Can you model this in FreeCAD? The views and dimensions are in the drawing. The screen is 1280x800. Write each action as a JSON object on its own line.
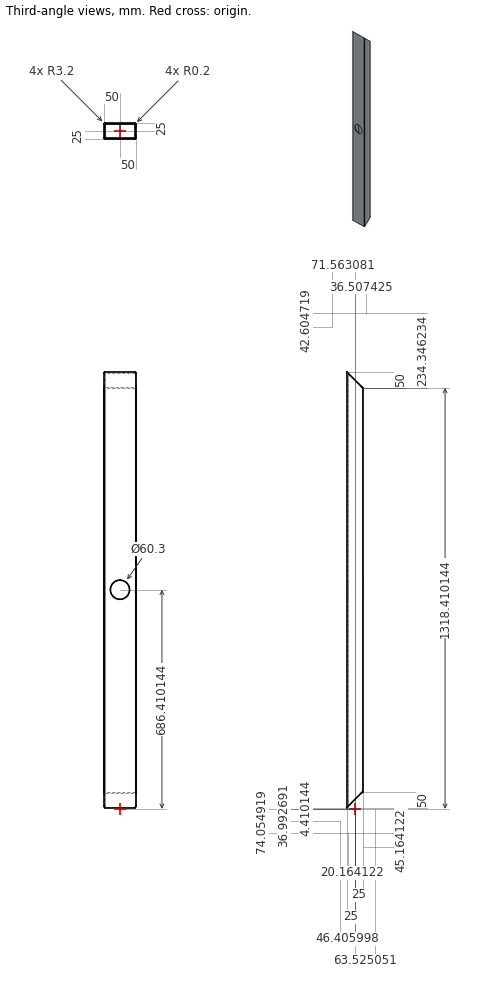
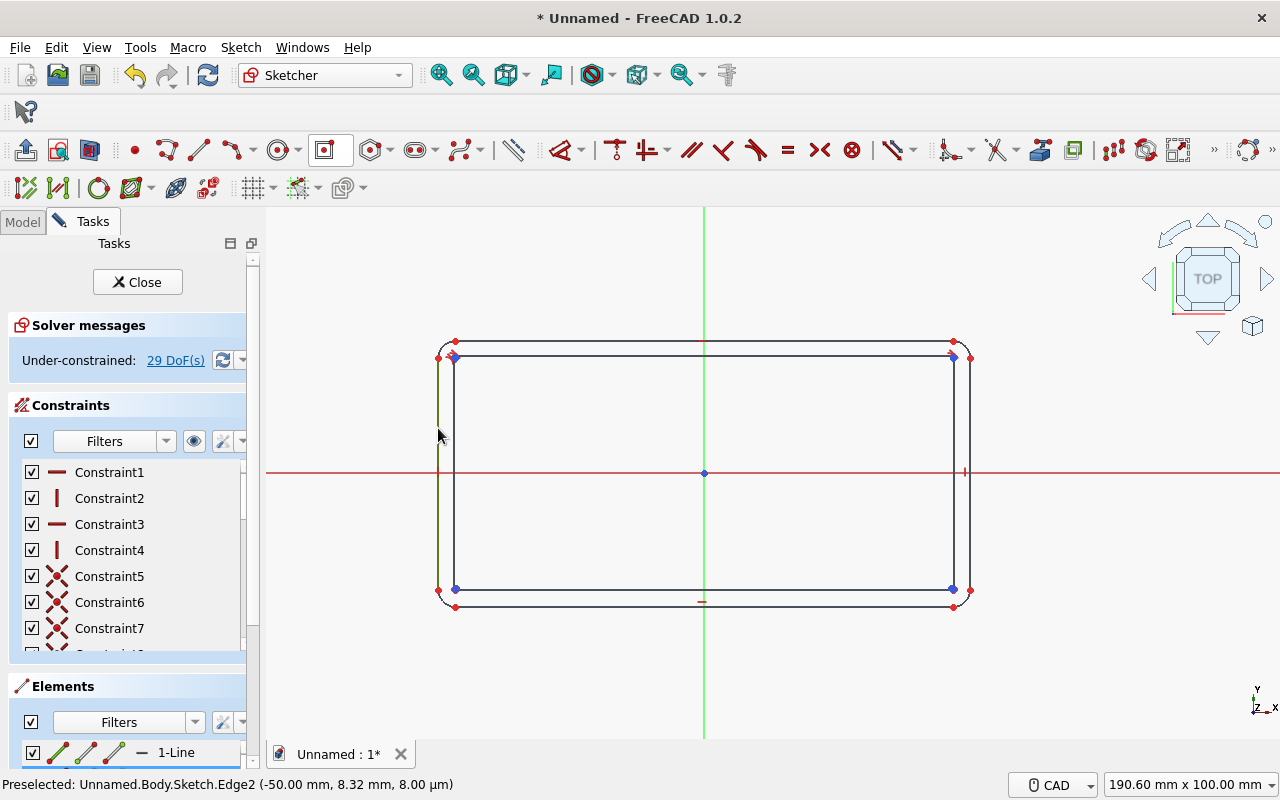
{"action": "left_click", "coordinate": [444, 602]}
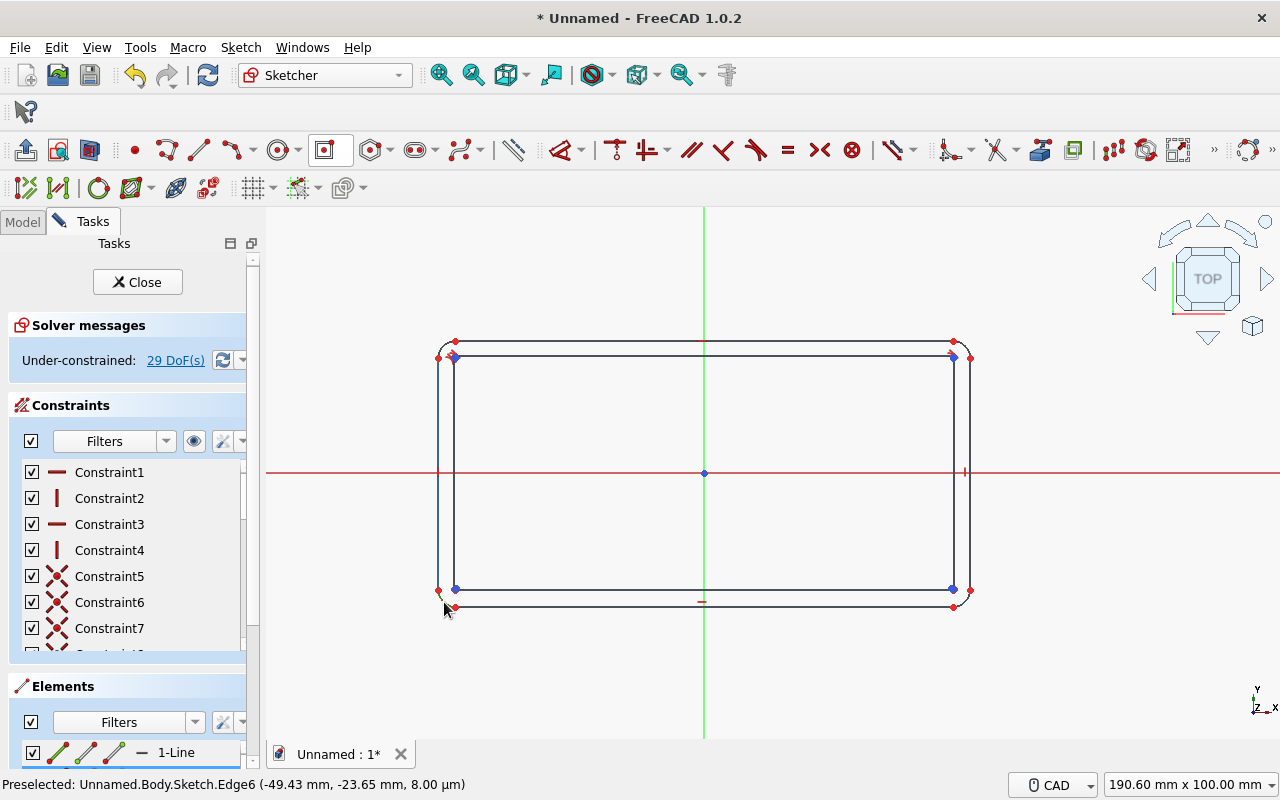
{"action": "left_click", "coordinate": [756, 150]}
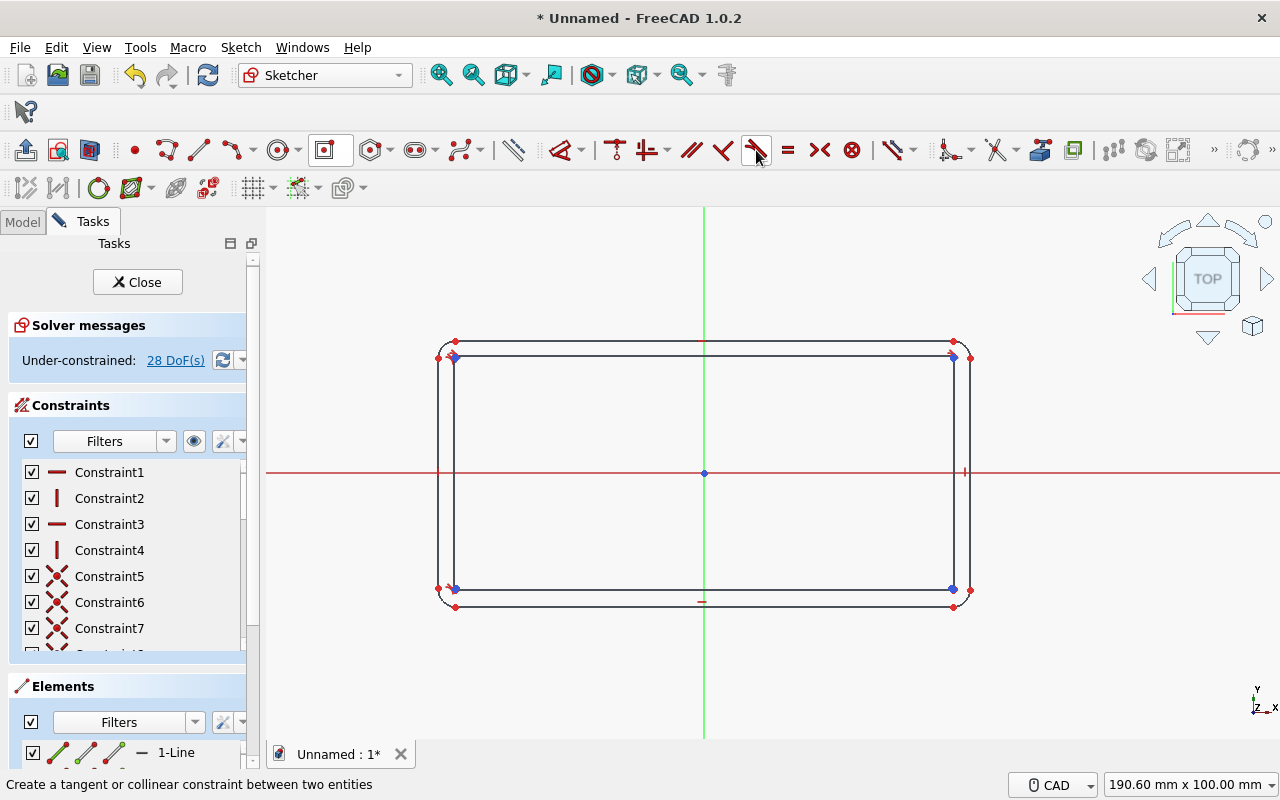
{"action": "left_click", "coordinate": [605, 607]}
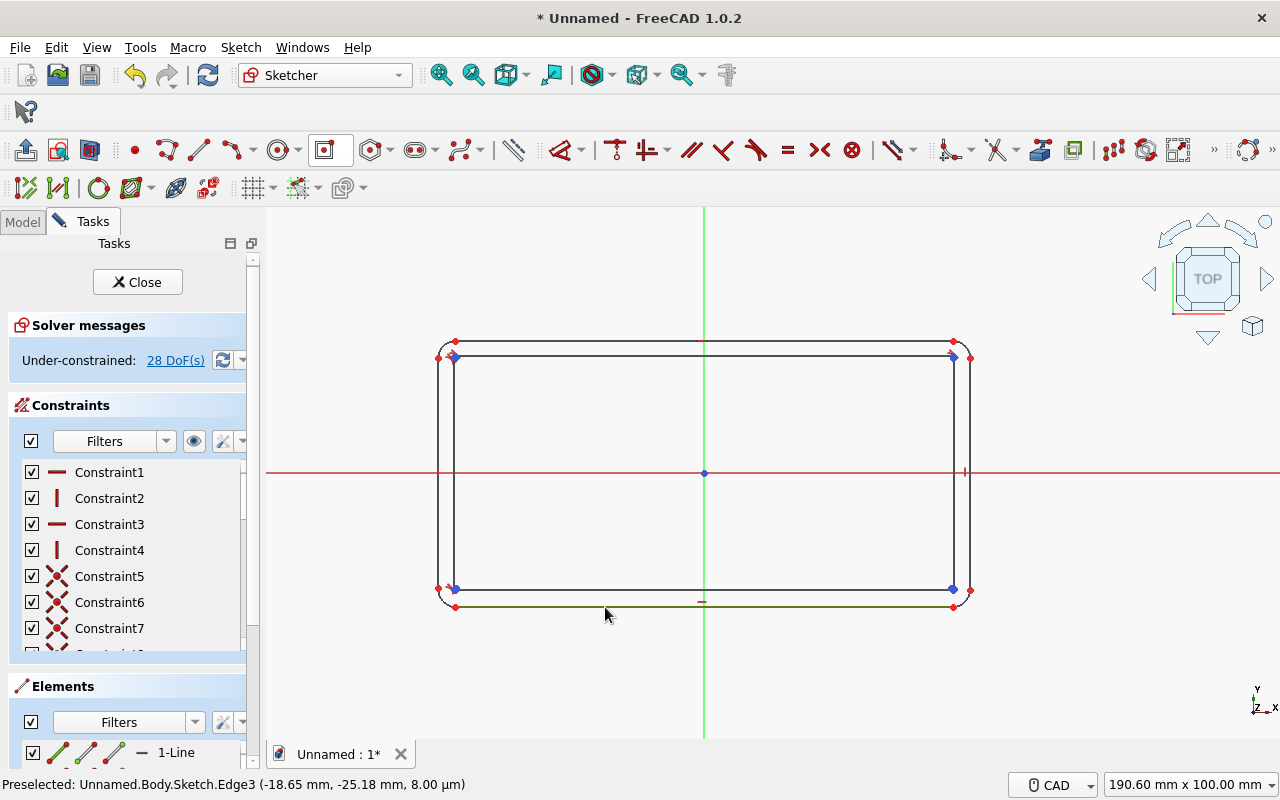
{"action": "left_click", "coordinate": [443, 601]}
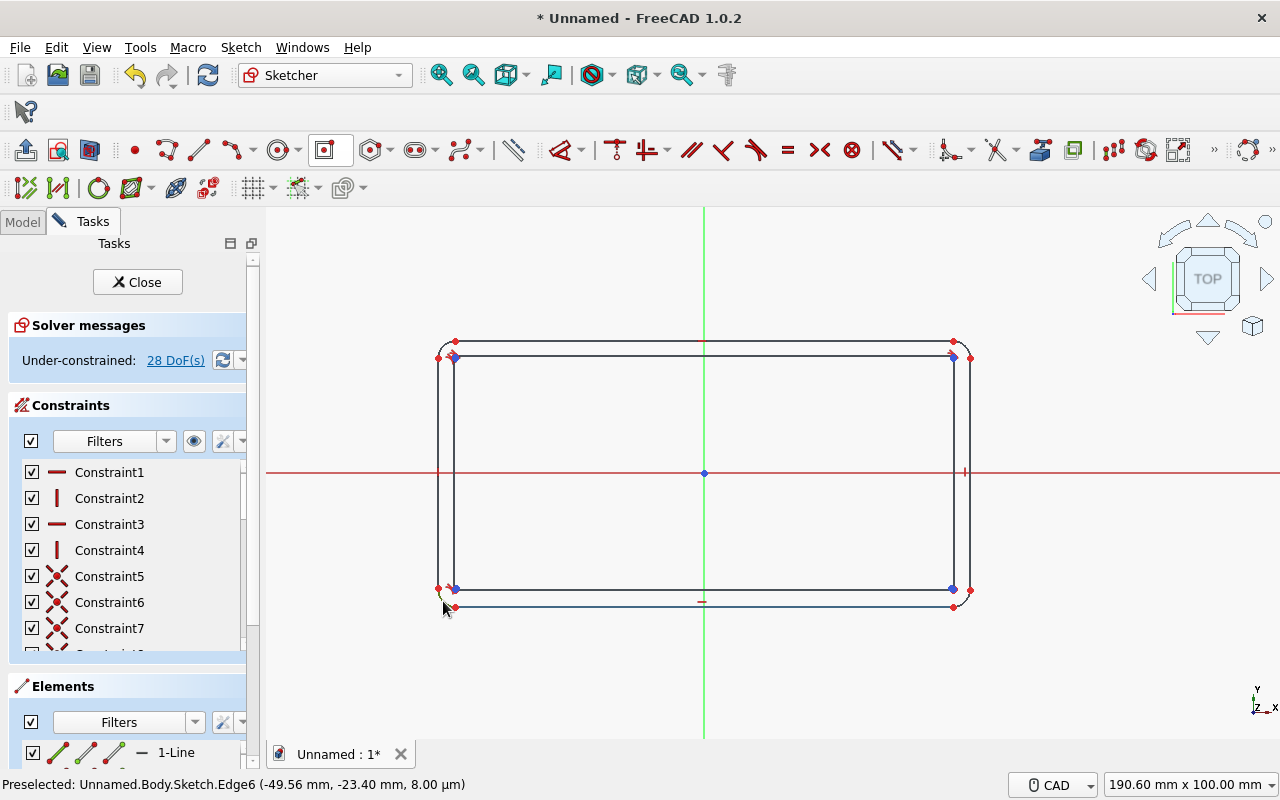
{"action": "left_click", "coordinate": [756, 150]}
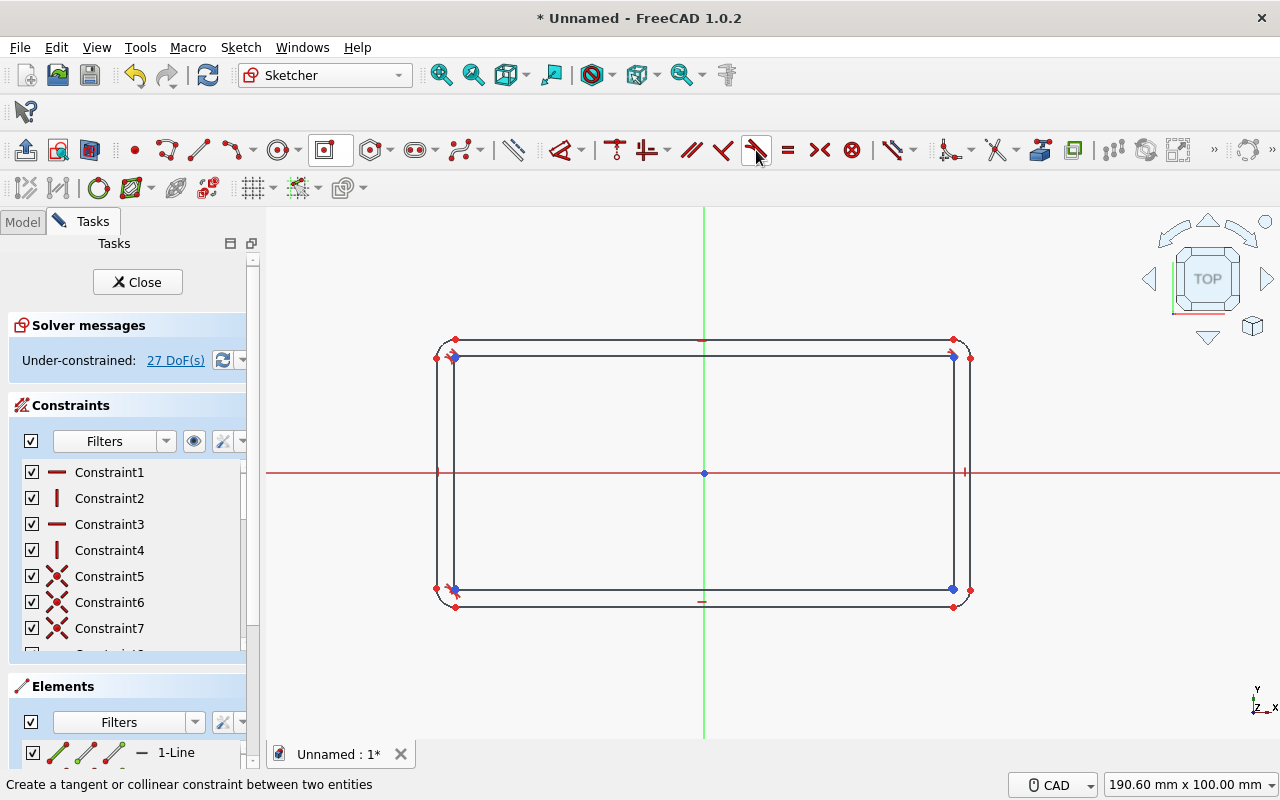
{"action": "left_click", "coordinate": [605, 607]}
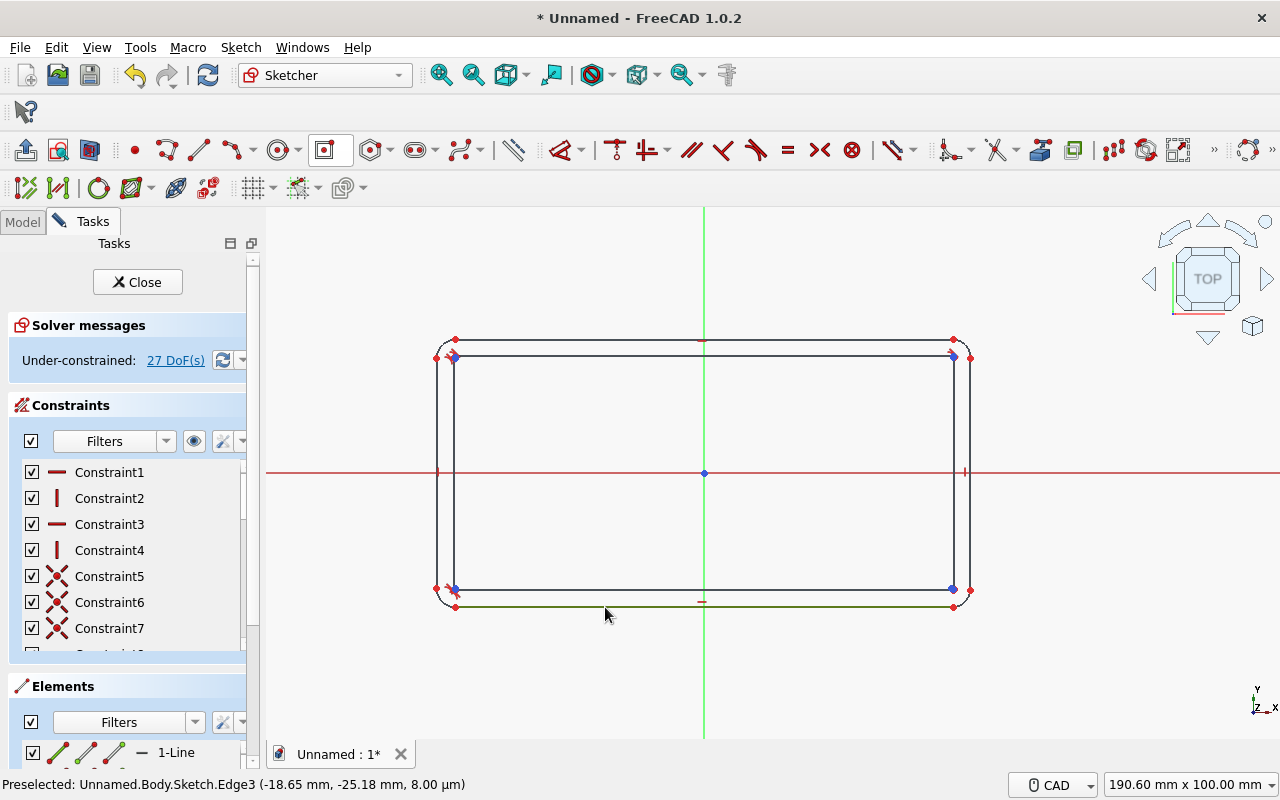
{"action": "left_click", "coordinate": [965, 602]}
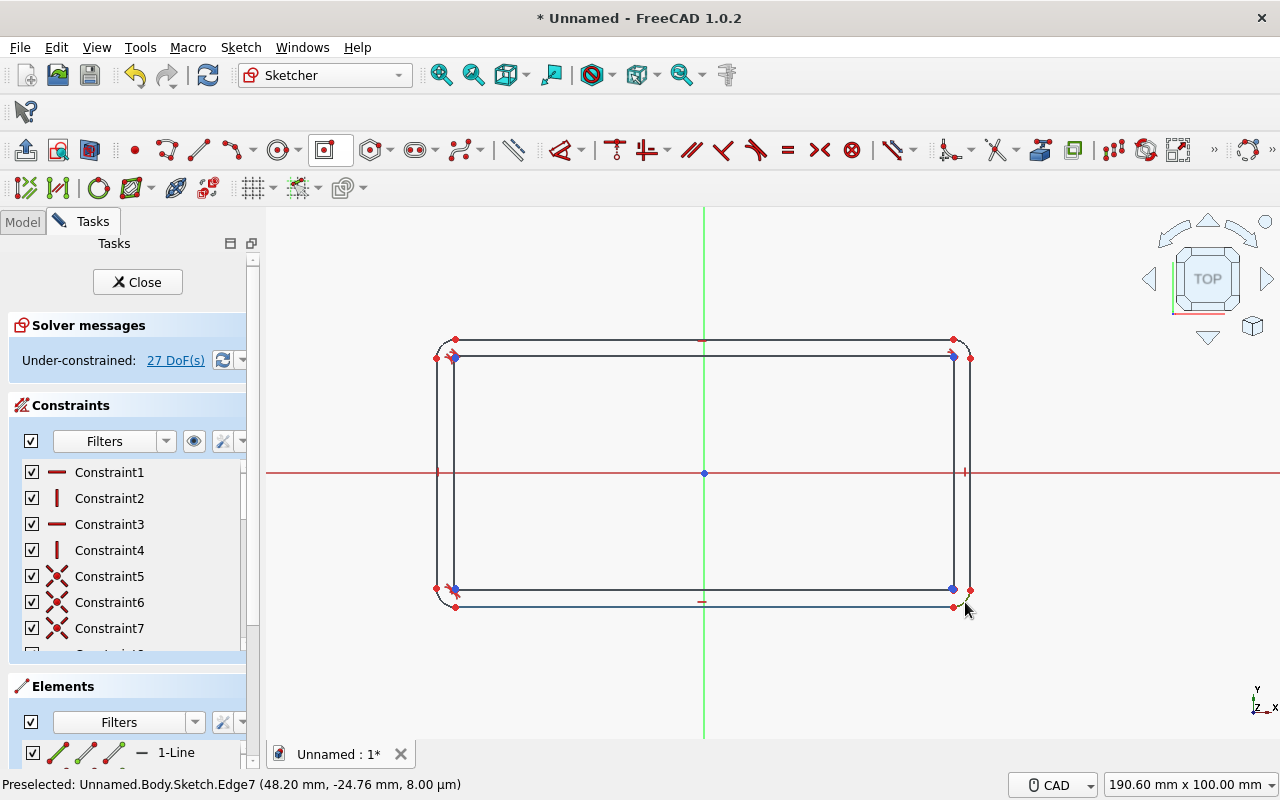
{"action": "left_click", "coordinate": [756, 150]}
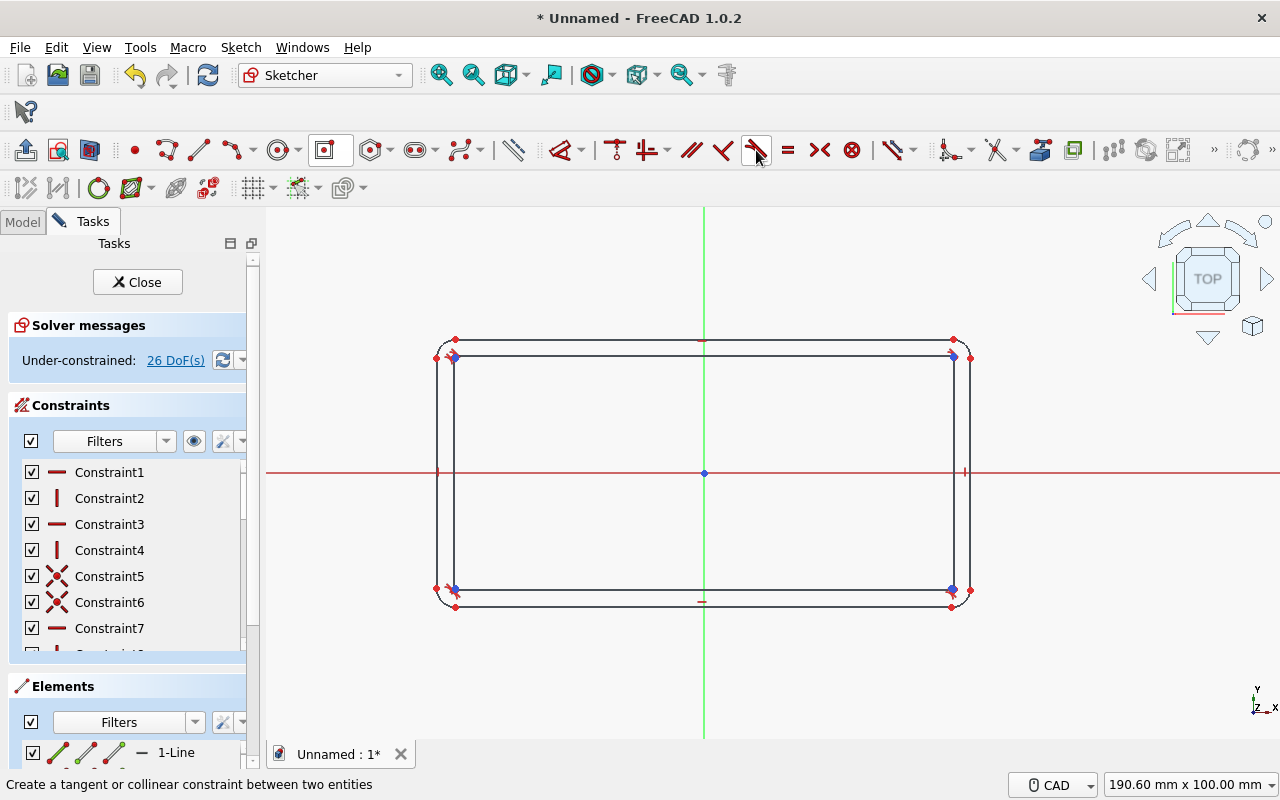
{"action": "left_click", "coordinate": [970, 521]}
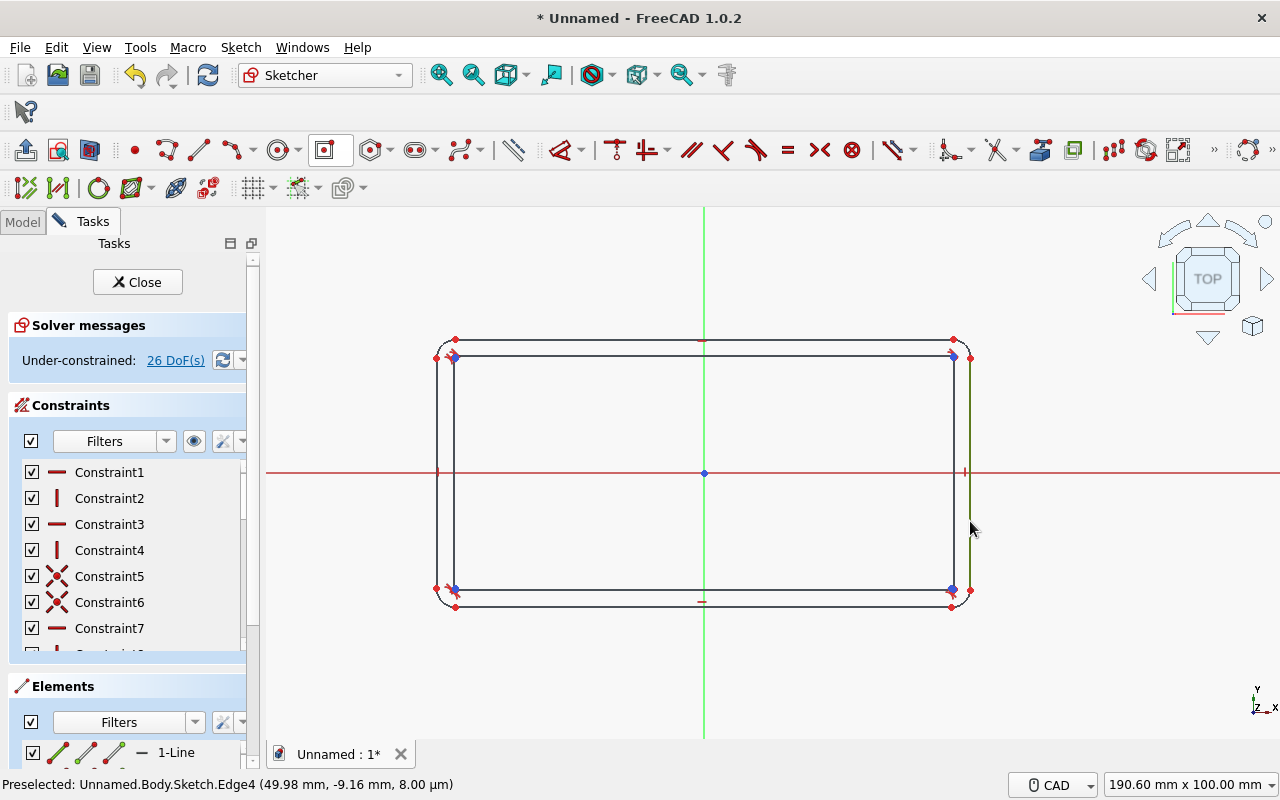
{"action": "left_click", "coordinate": [964, 602]}